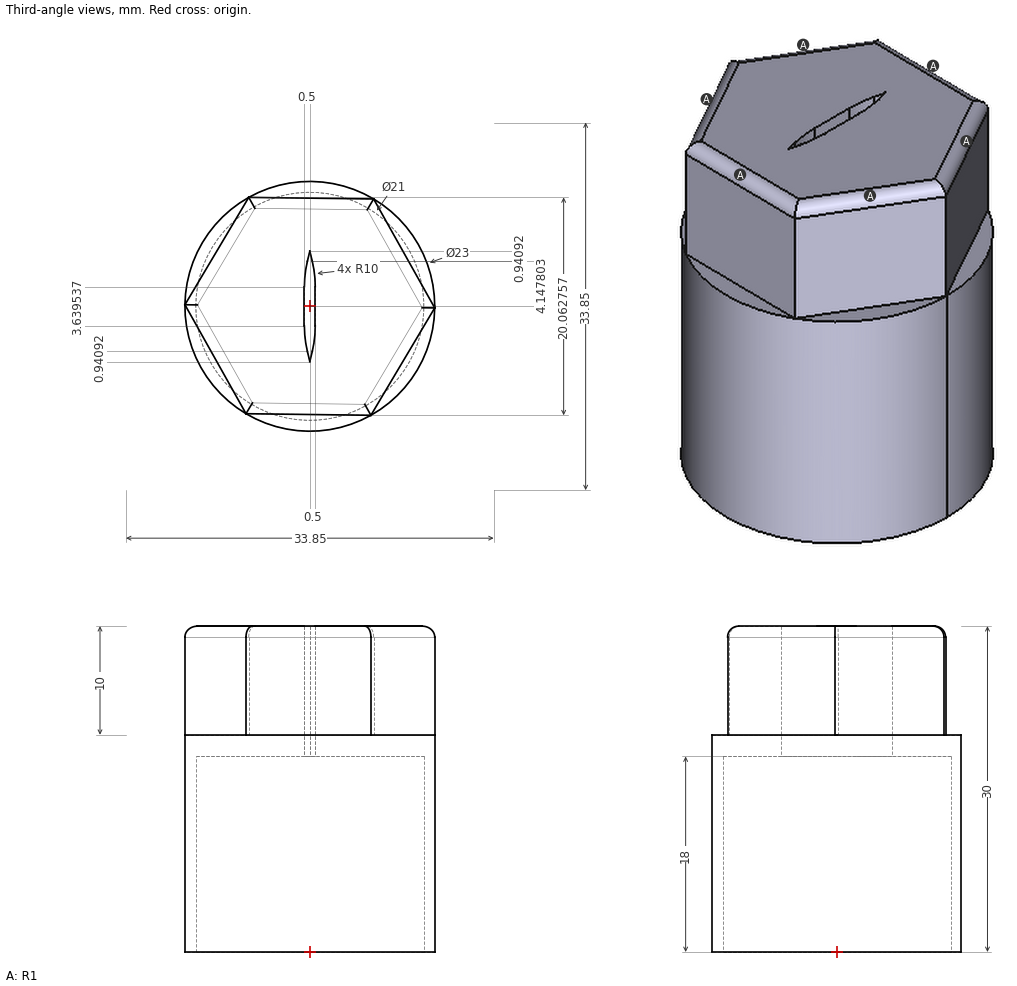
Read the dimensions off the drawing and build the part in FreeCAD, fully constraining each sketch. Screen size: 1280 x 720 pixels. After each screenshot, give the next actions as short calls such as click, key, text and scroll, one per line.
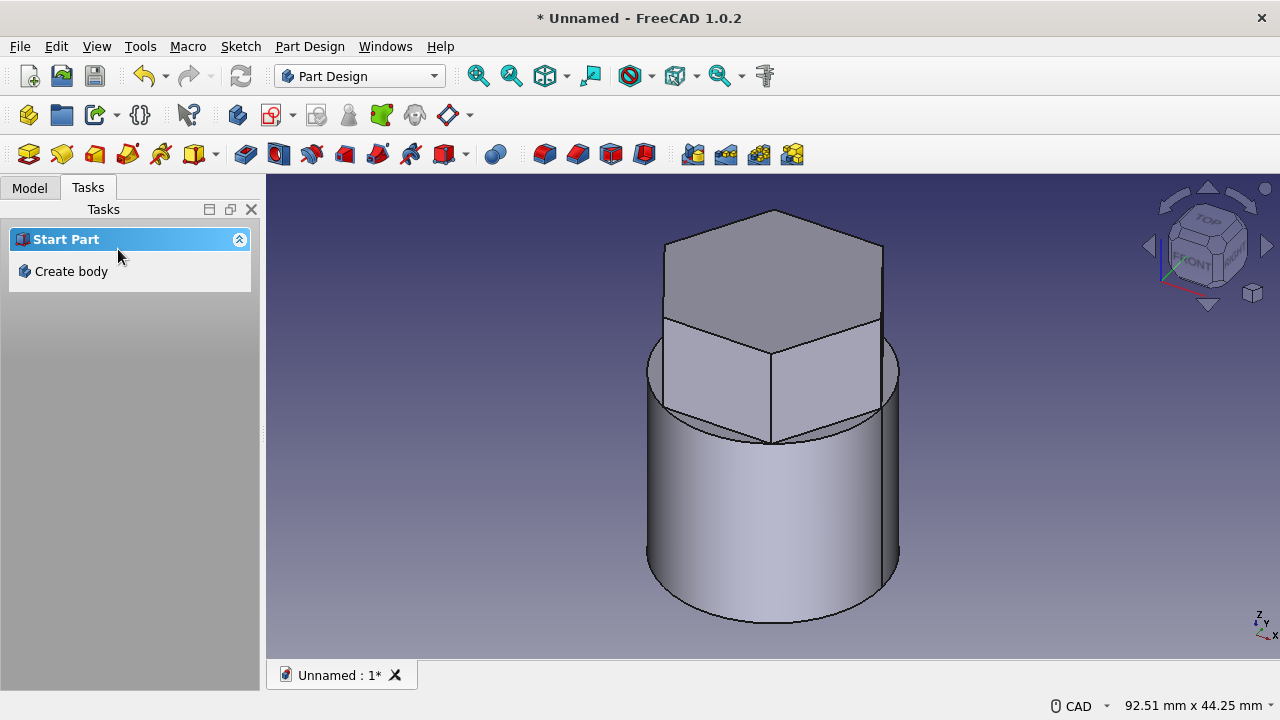
click(773, 281)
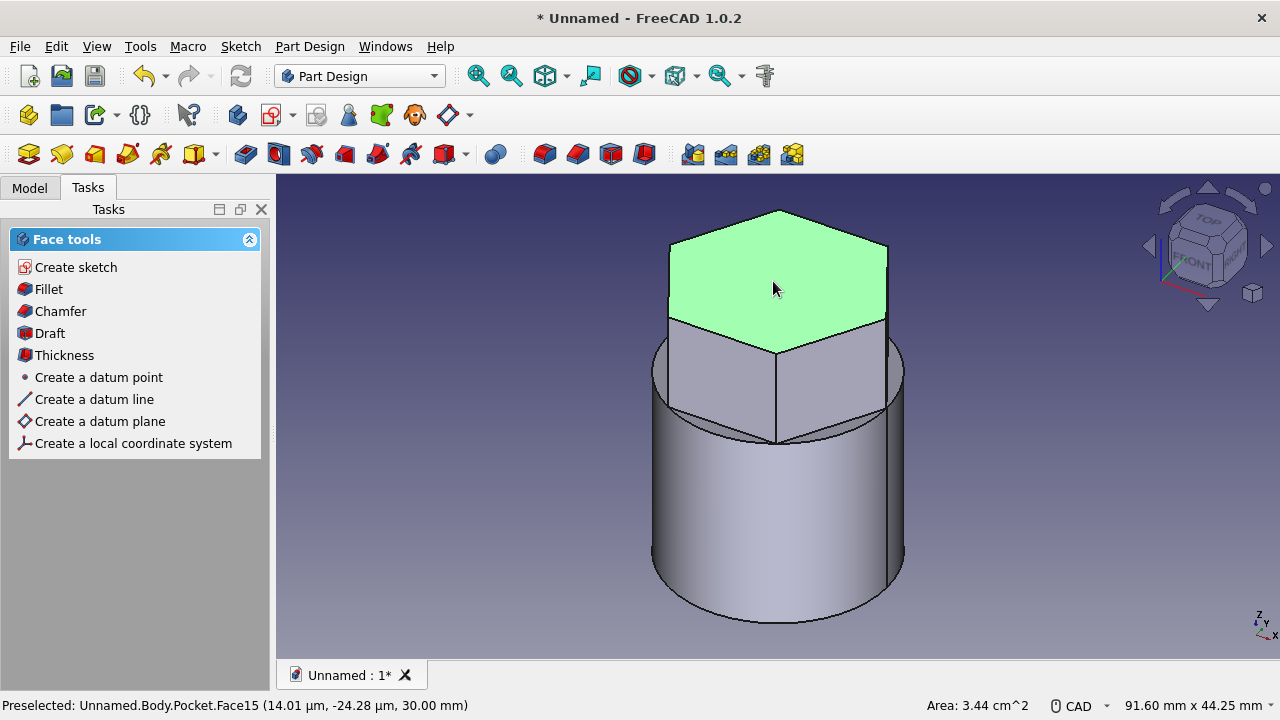
click(545, 154)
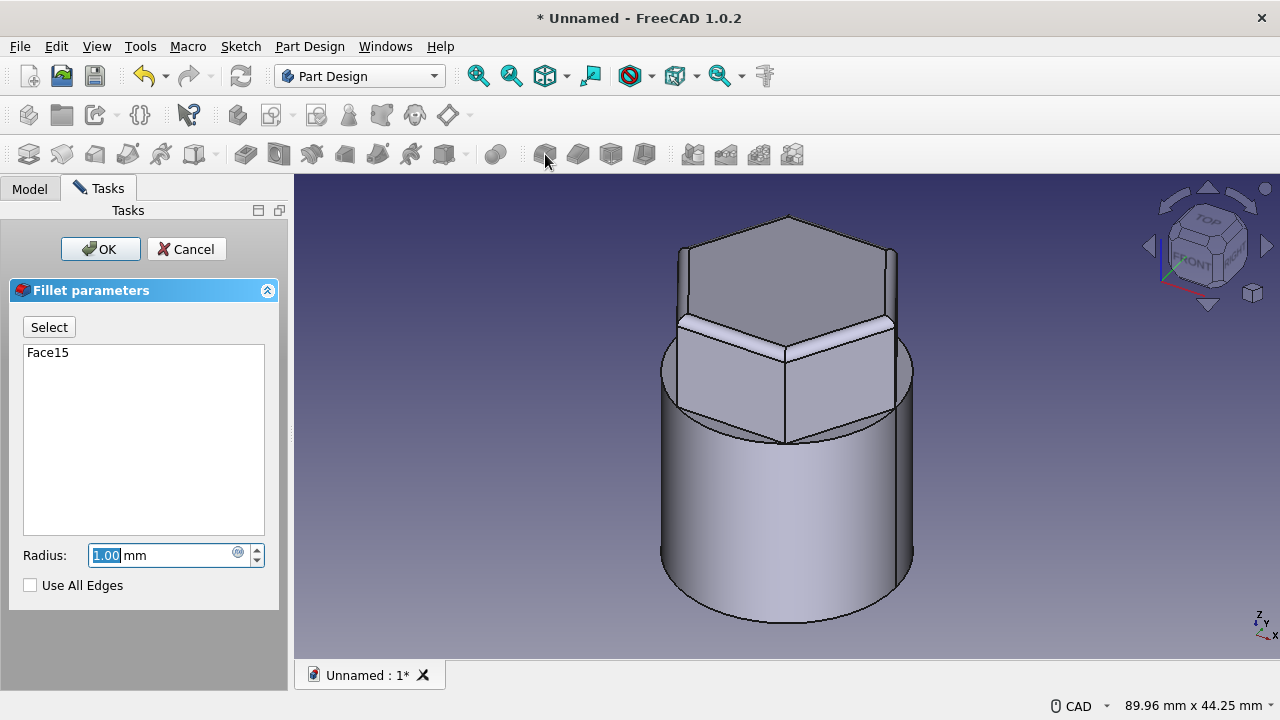
text(1)
key(Tab)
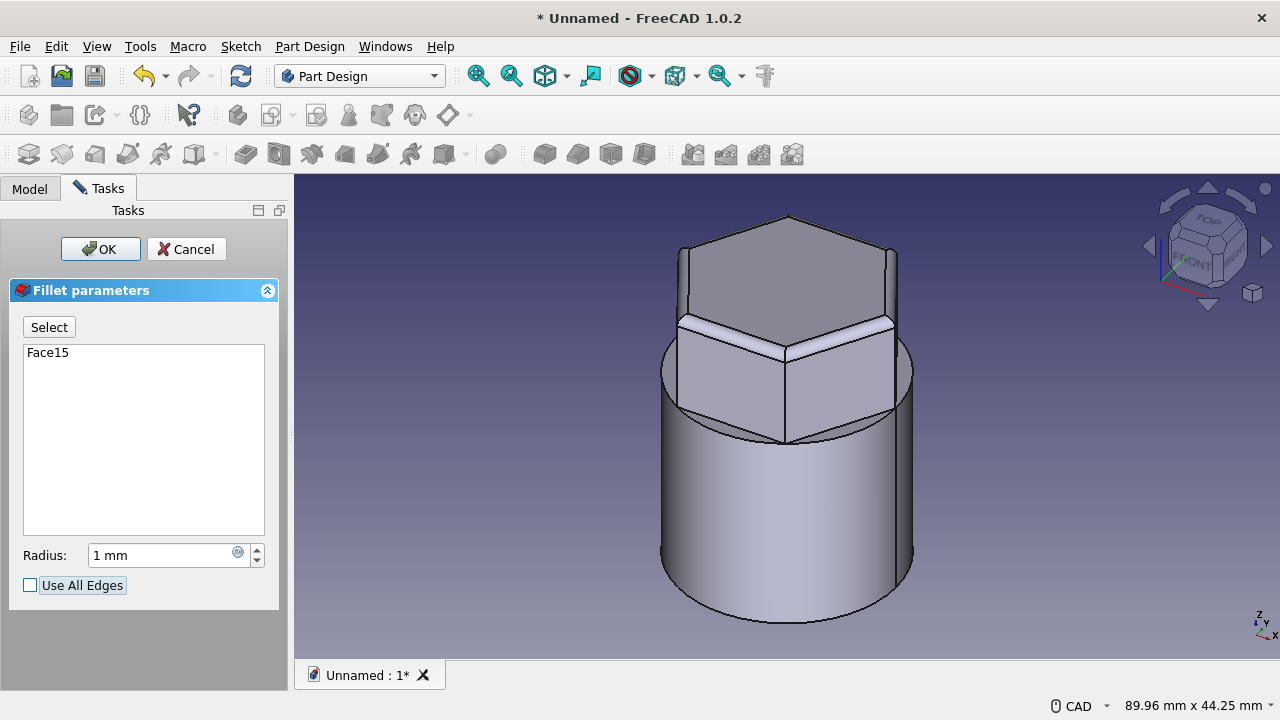
click(101, 249)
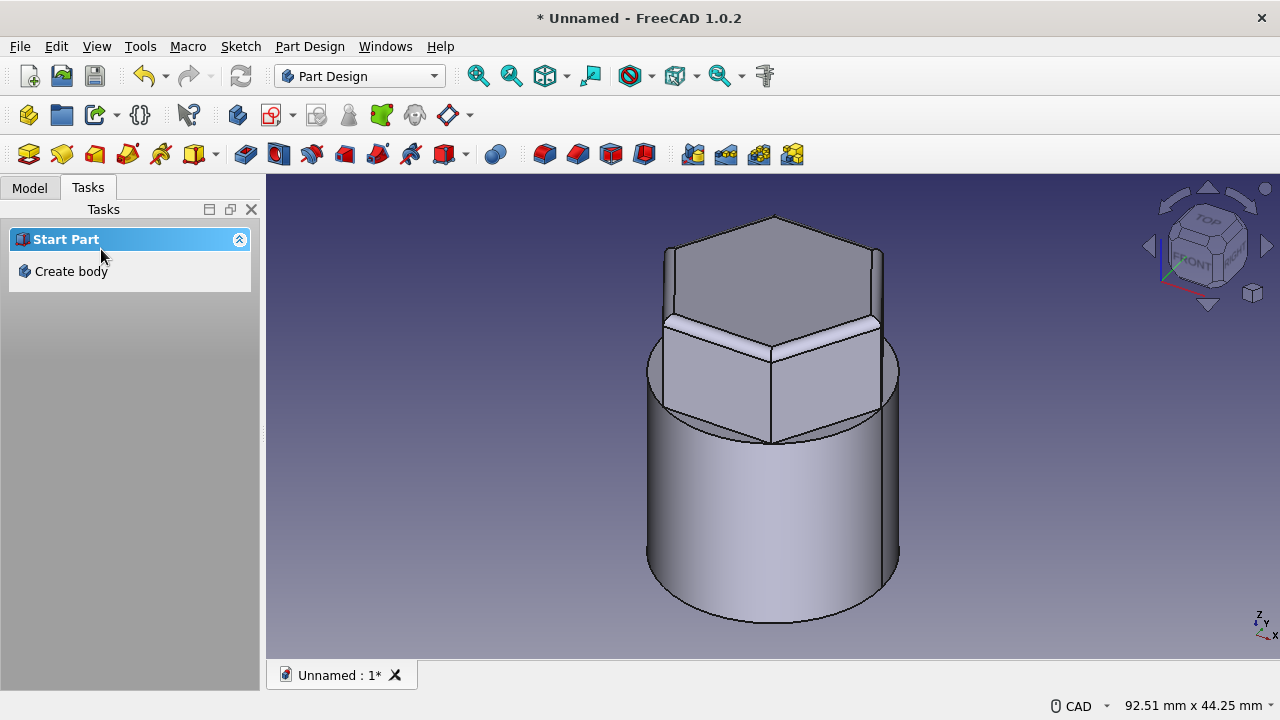
click(773, 281)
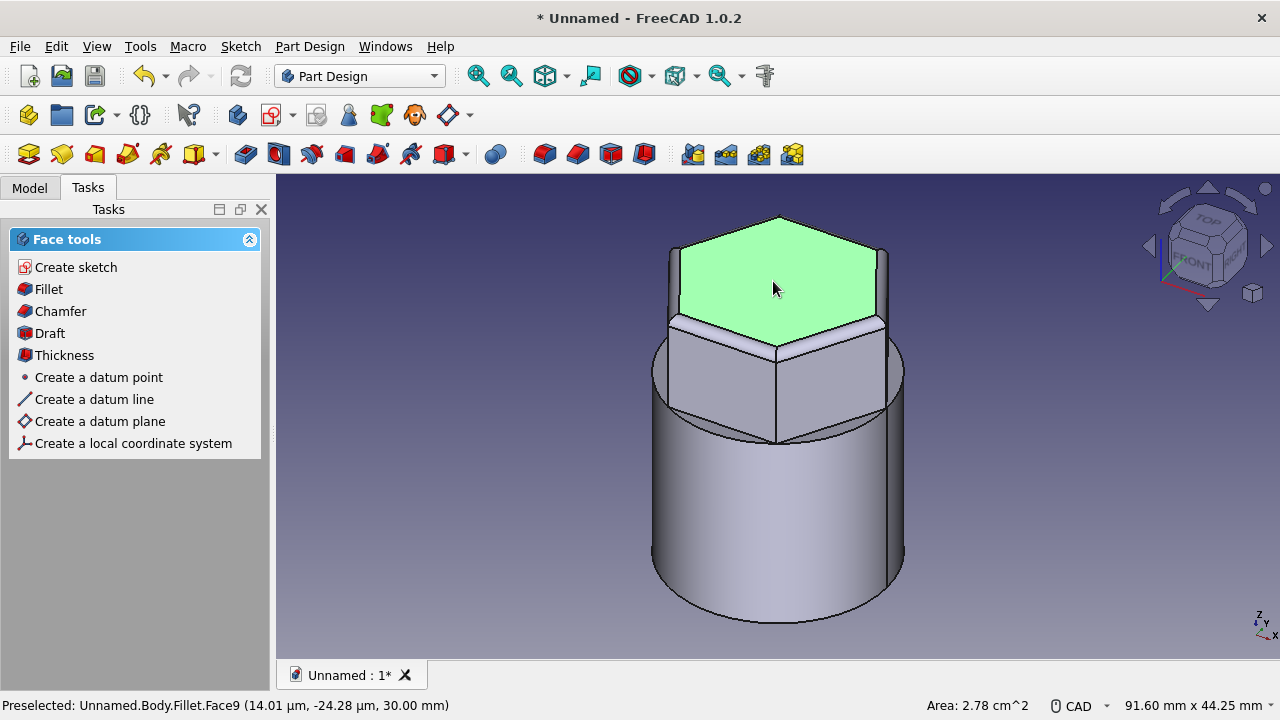
click(270, 116)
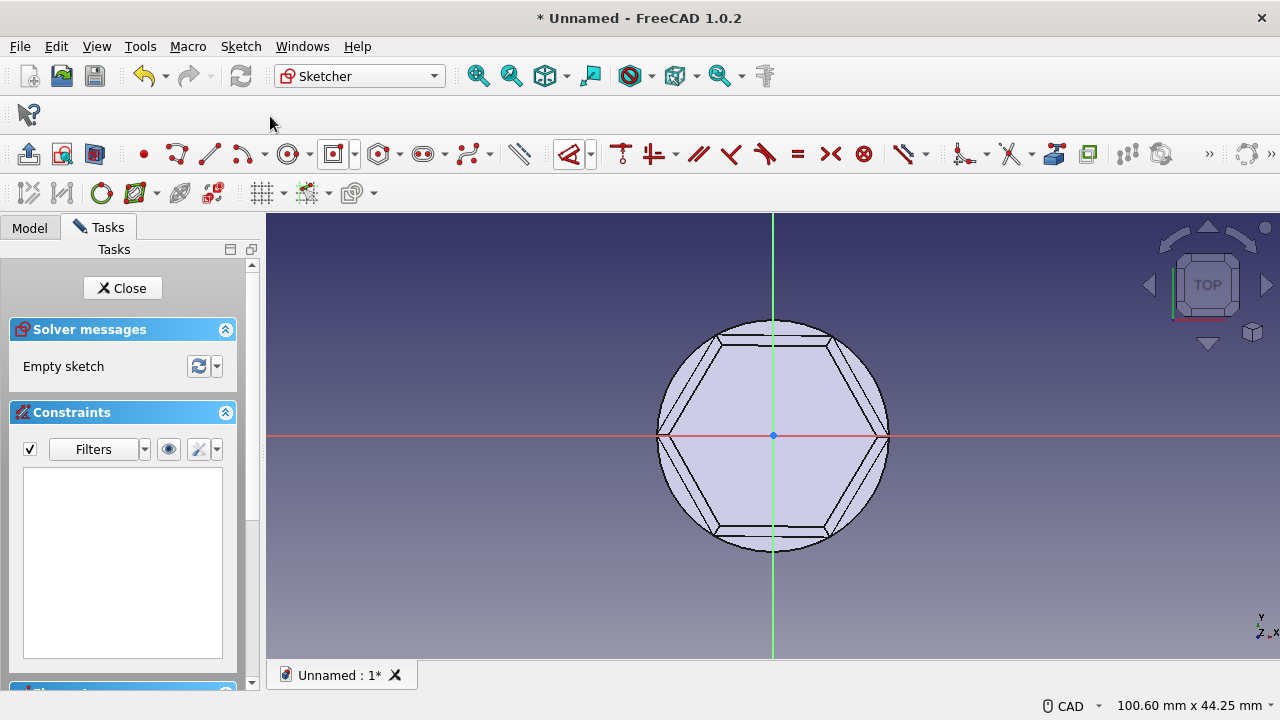
scroll(813, 436, up, 5)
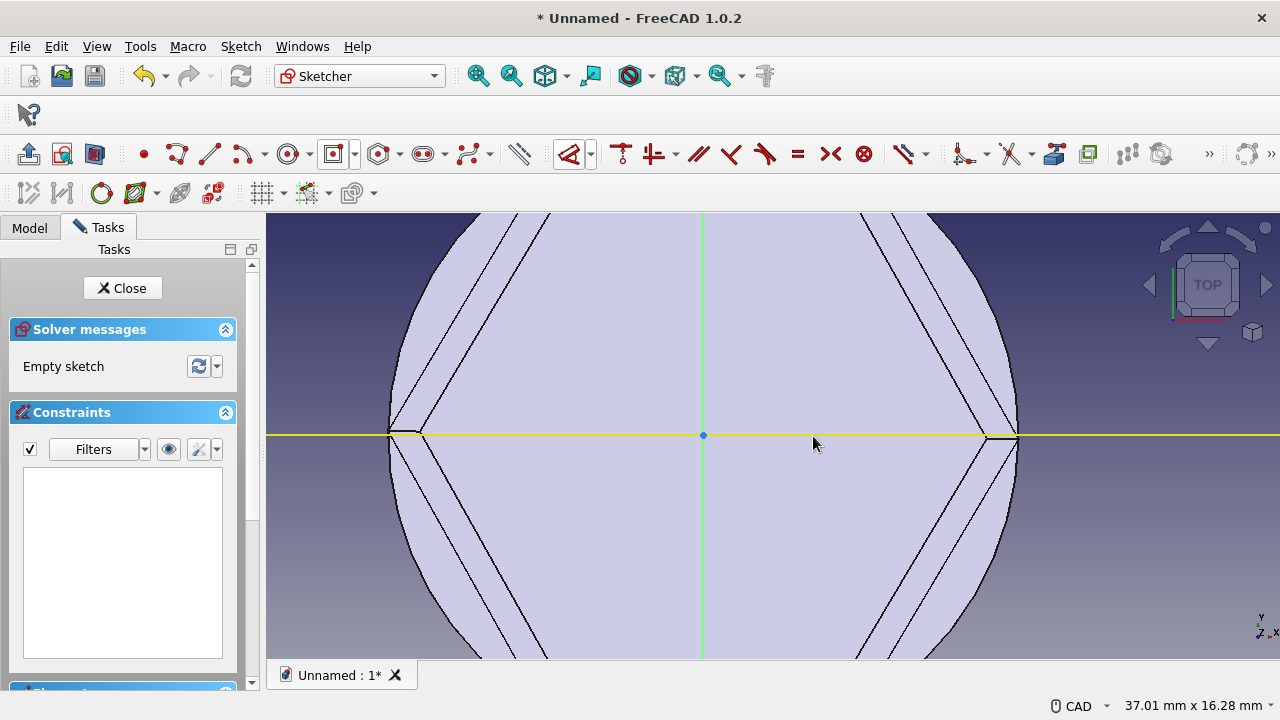
key(g)
key(m)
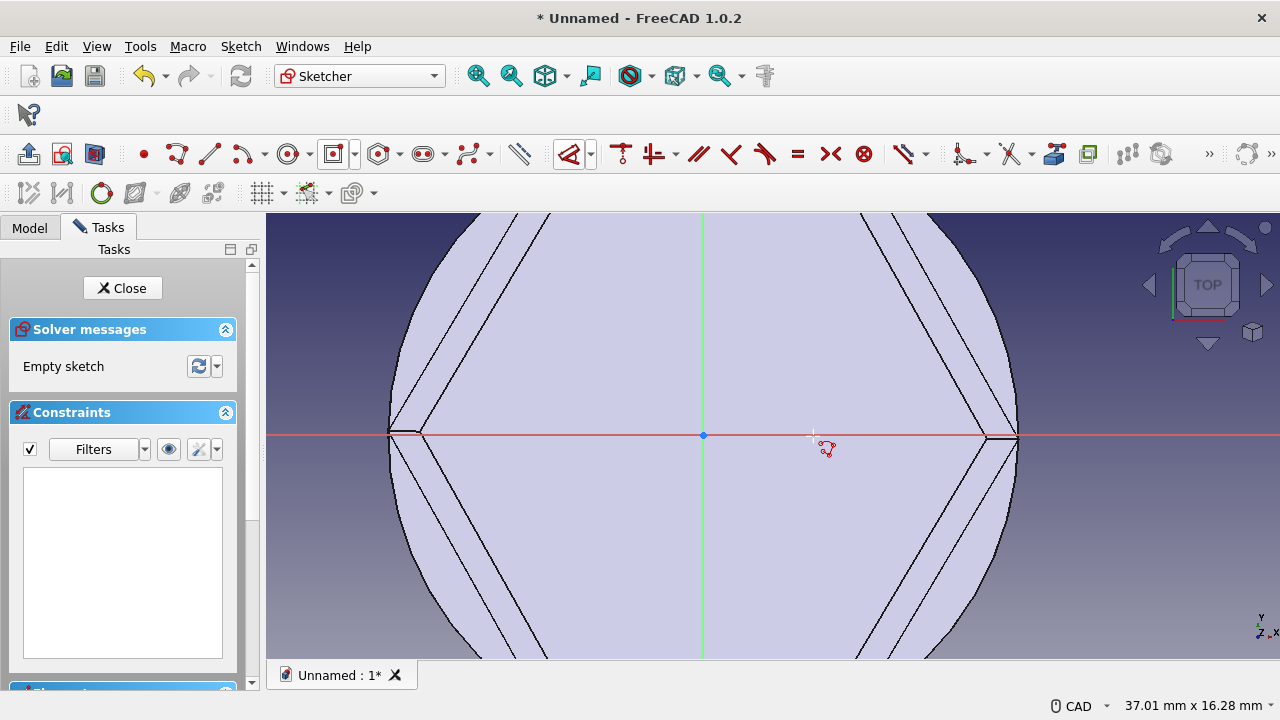
scroll(710, 321, up, 5)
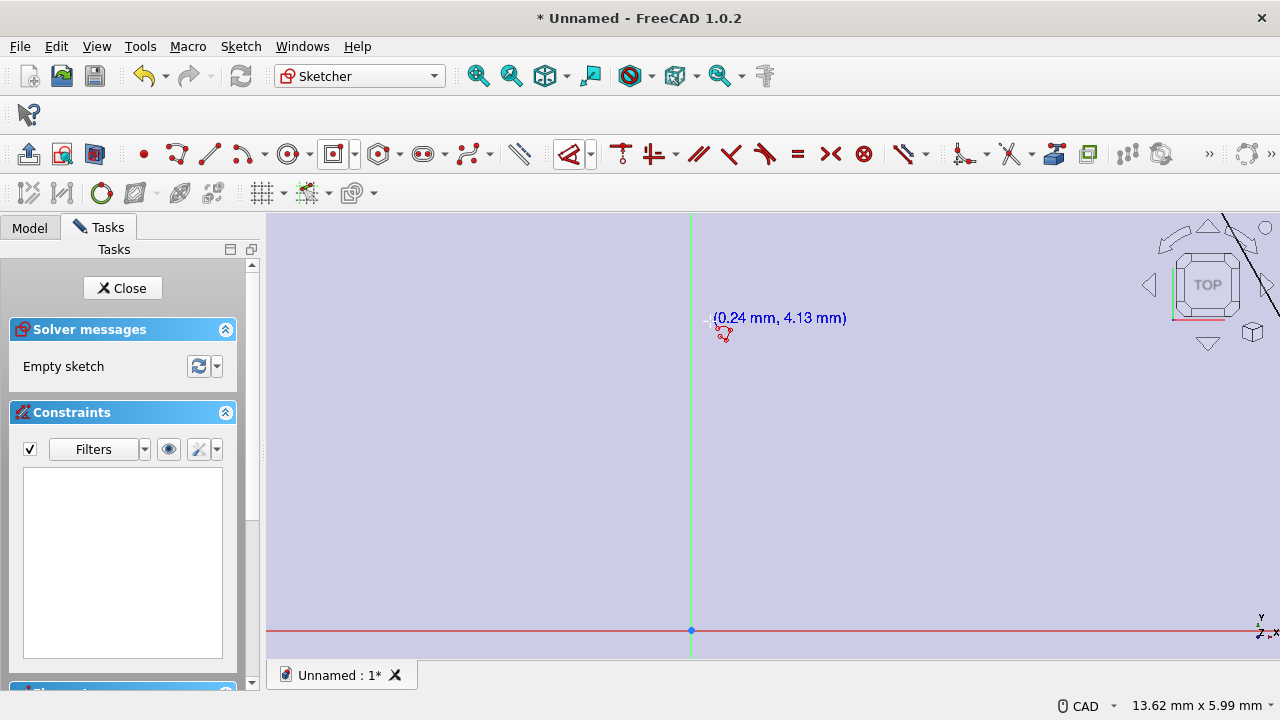
click(708, 322)
click(691, 252)
click(674, 322)
right_click(674, 322)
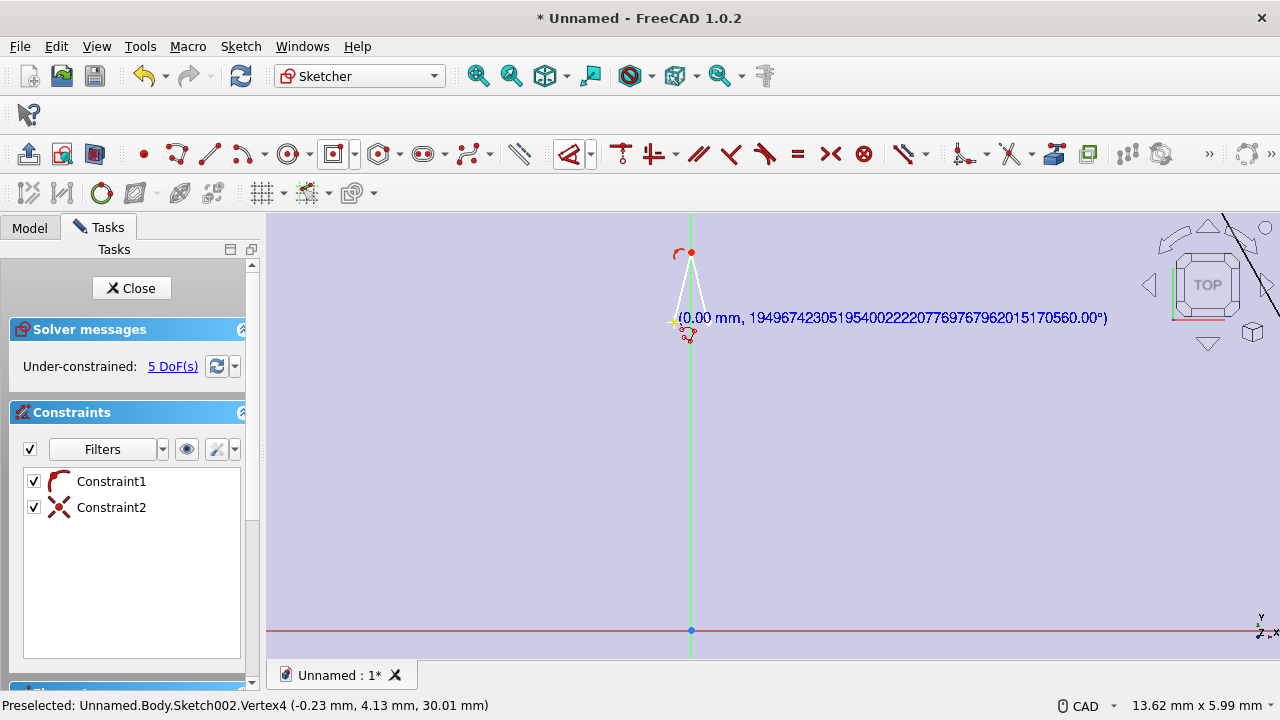
click(210, 154)